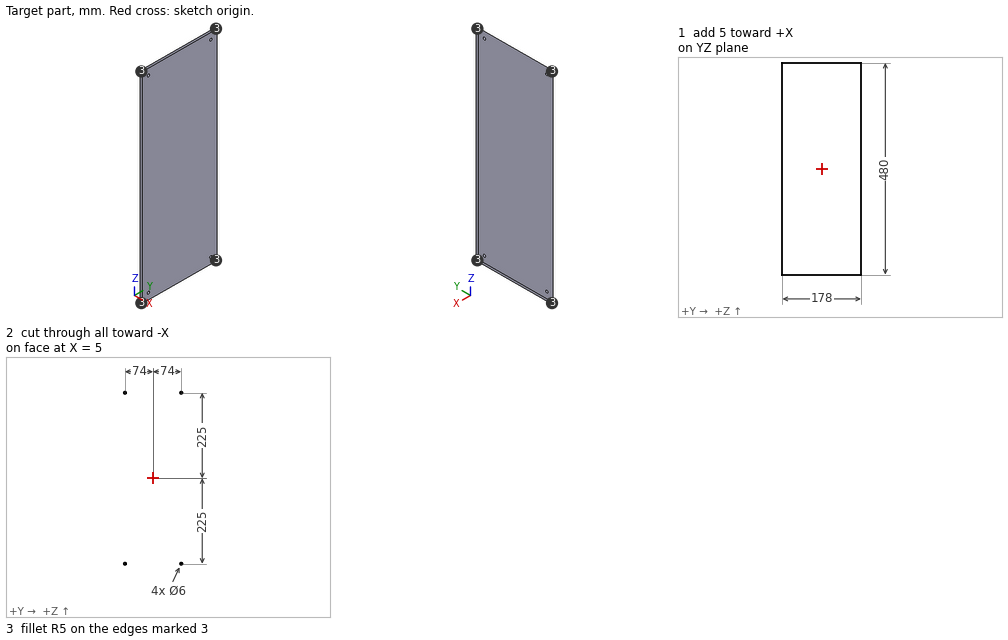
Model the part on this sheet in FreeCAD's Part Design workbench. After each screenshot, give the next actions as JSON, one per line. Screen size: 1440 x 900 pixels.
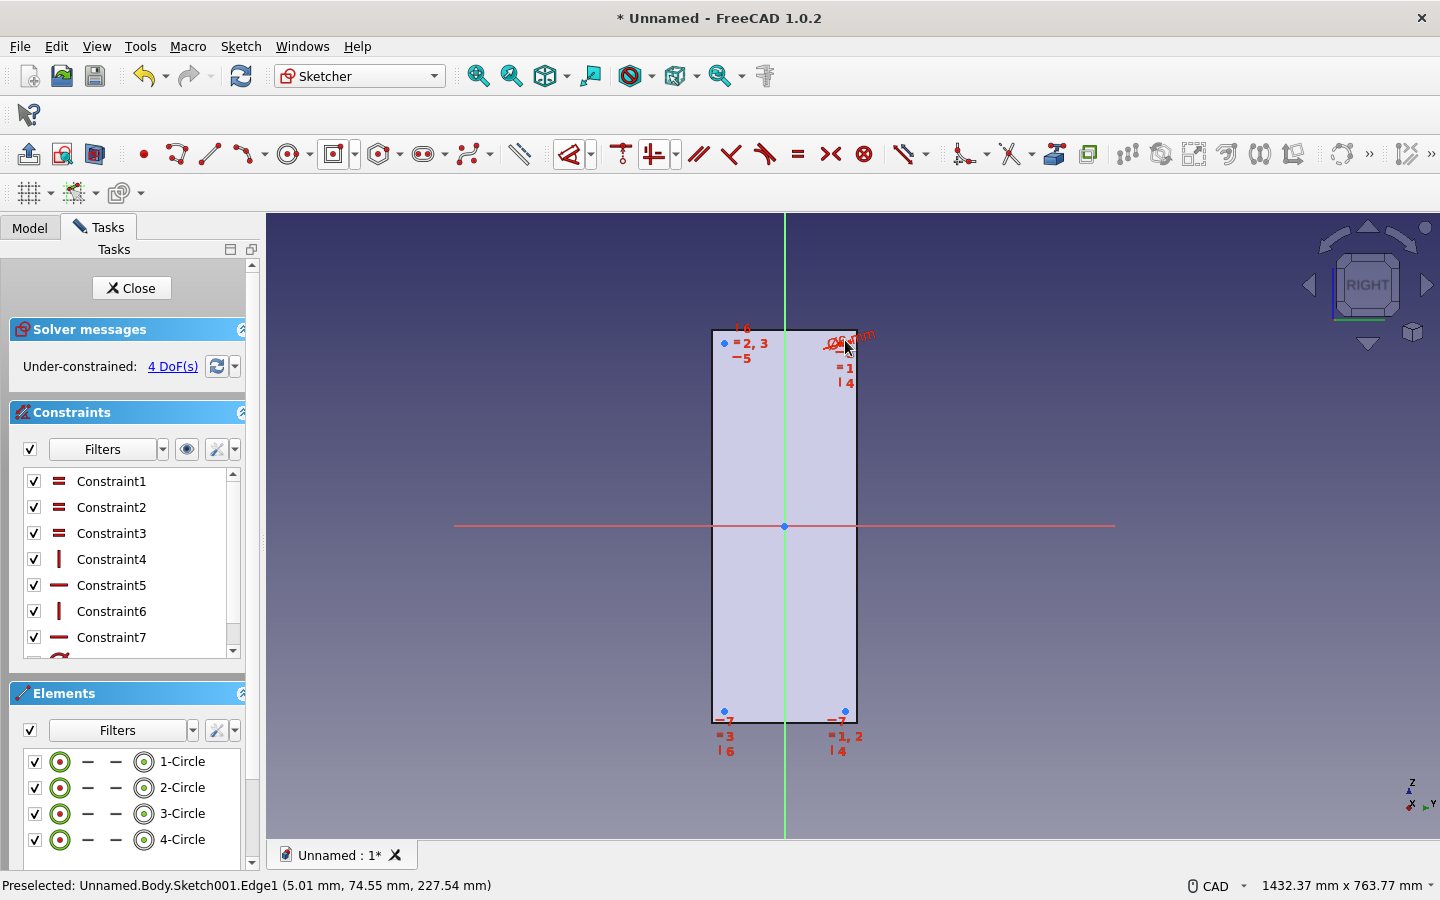
{"action": "left_click", "coordinate": [845, 343]}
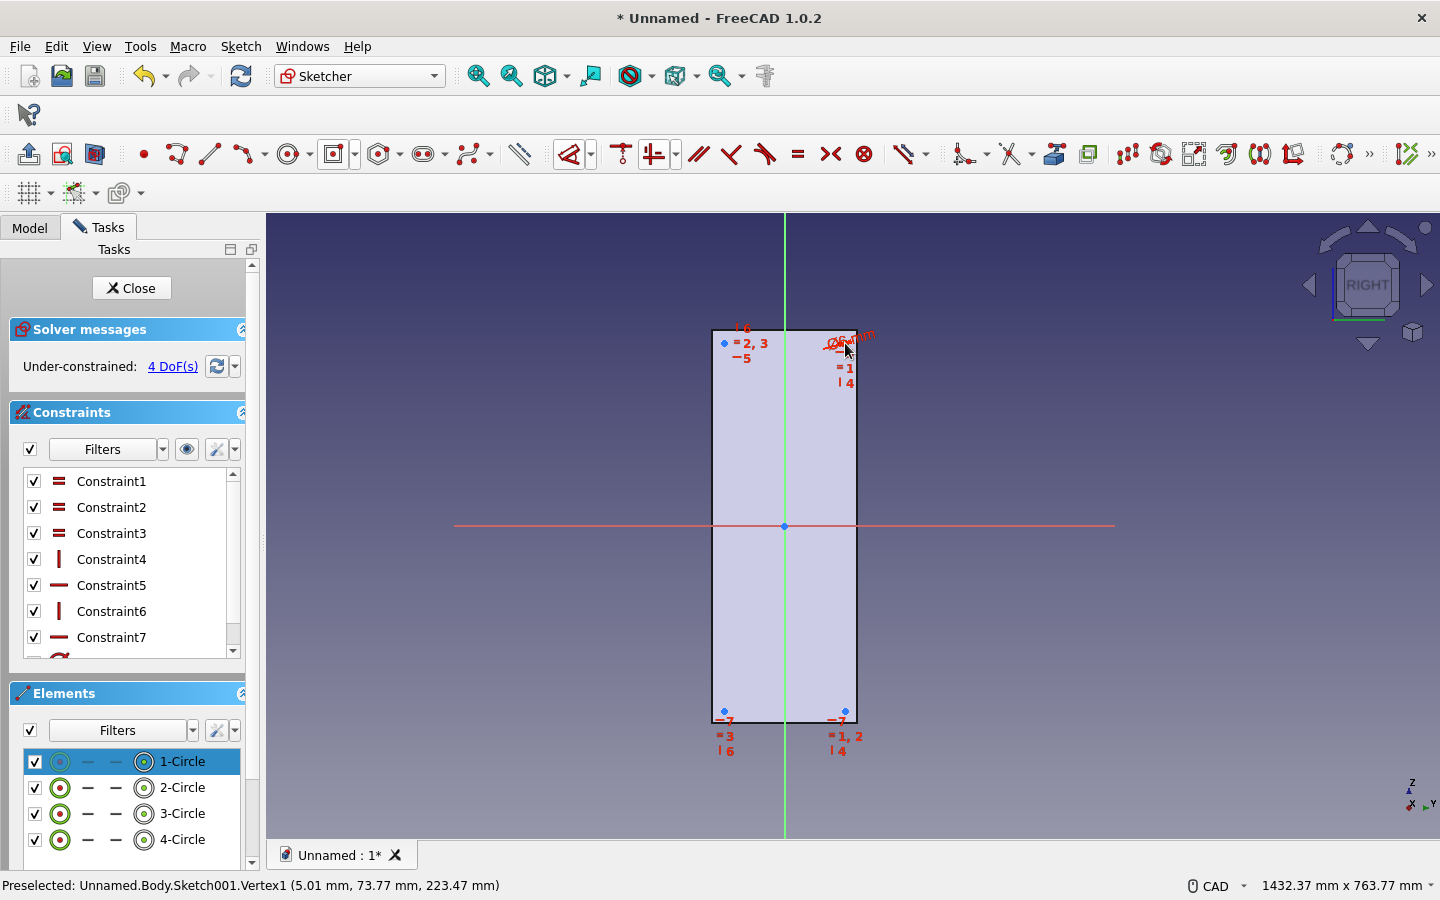
{"action": "left_click", "coordinate": [590, 154]}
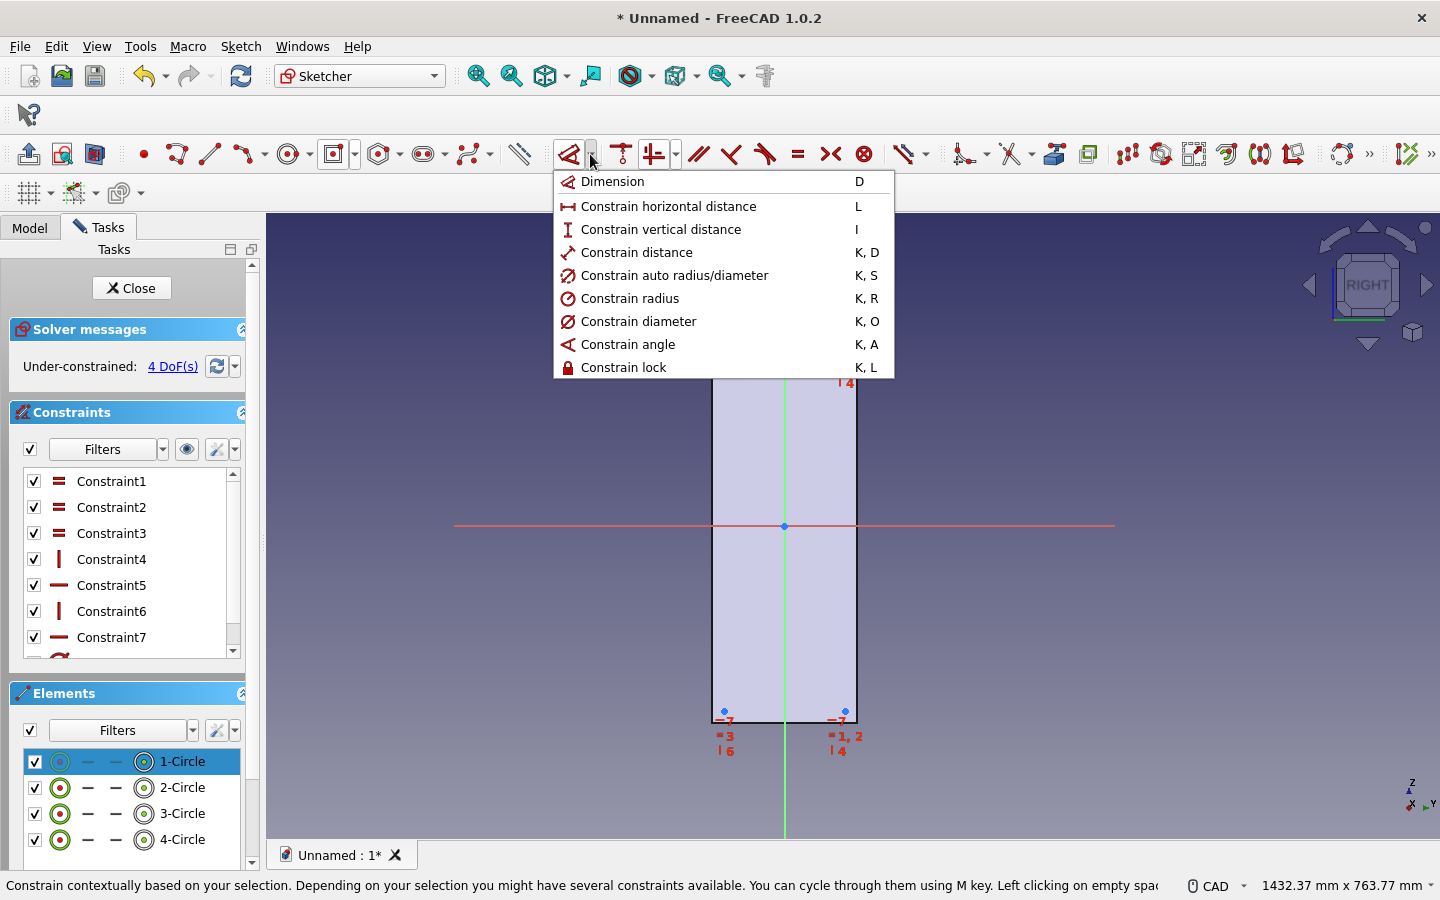
{"action": "left_click", "coordinate": [724, 206]}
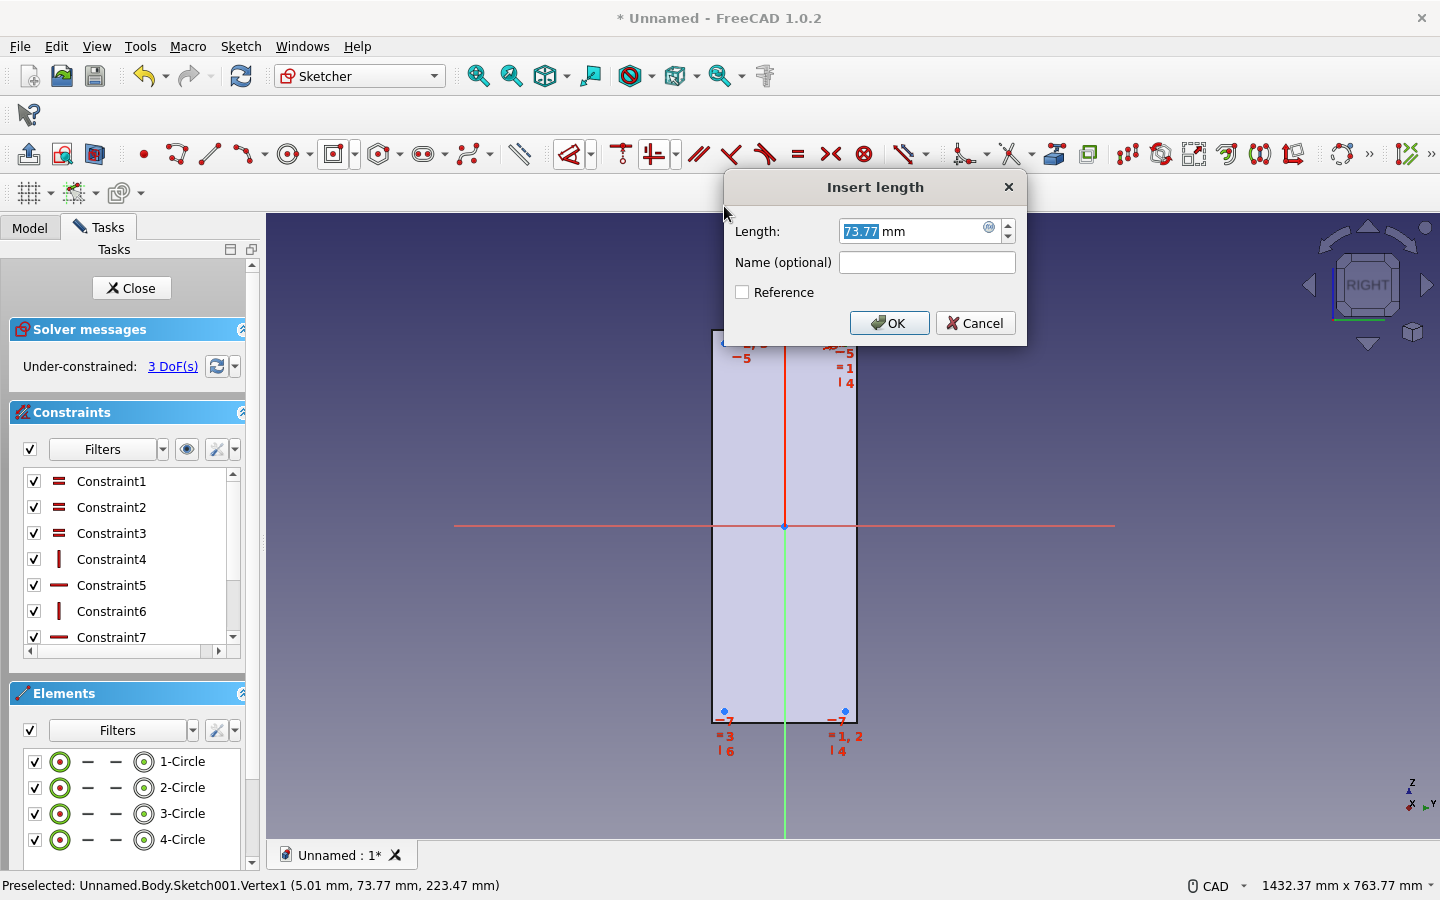
{"action": "type", "text": "74"}
{"action": "key", "text": "Return"}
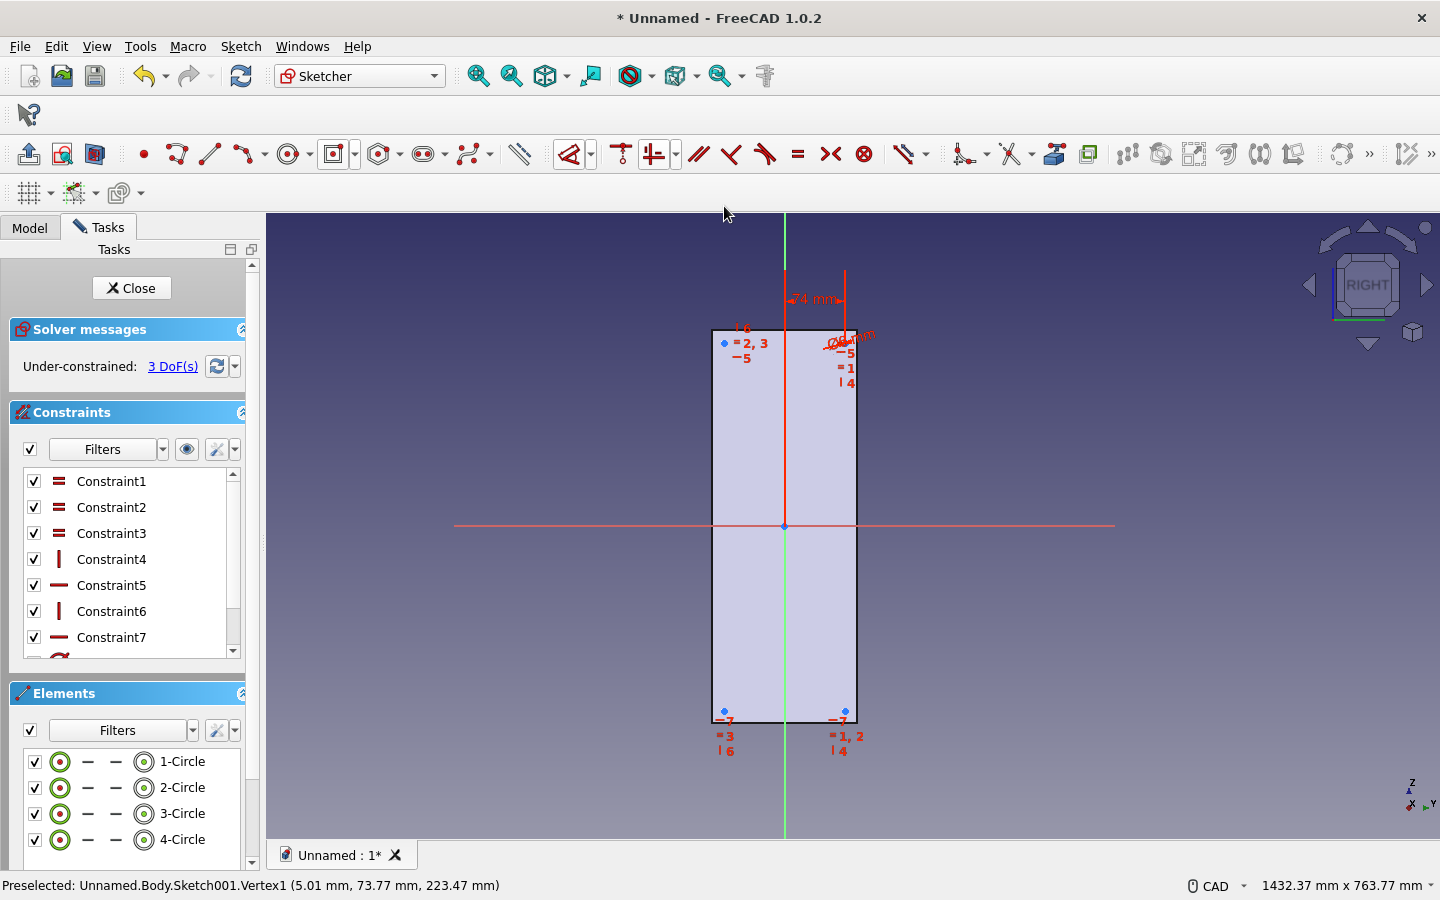
{"action": "left_click", "coordinate": [724, 343]}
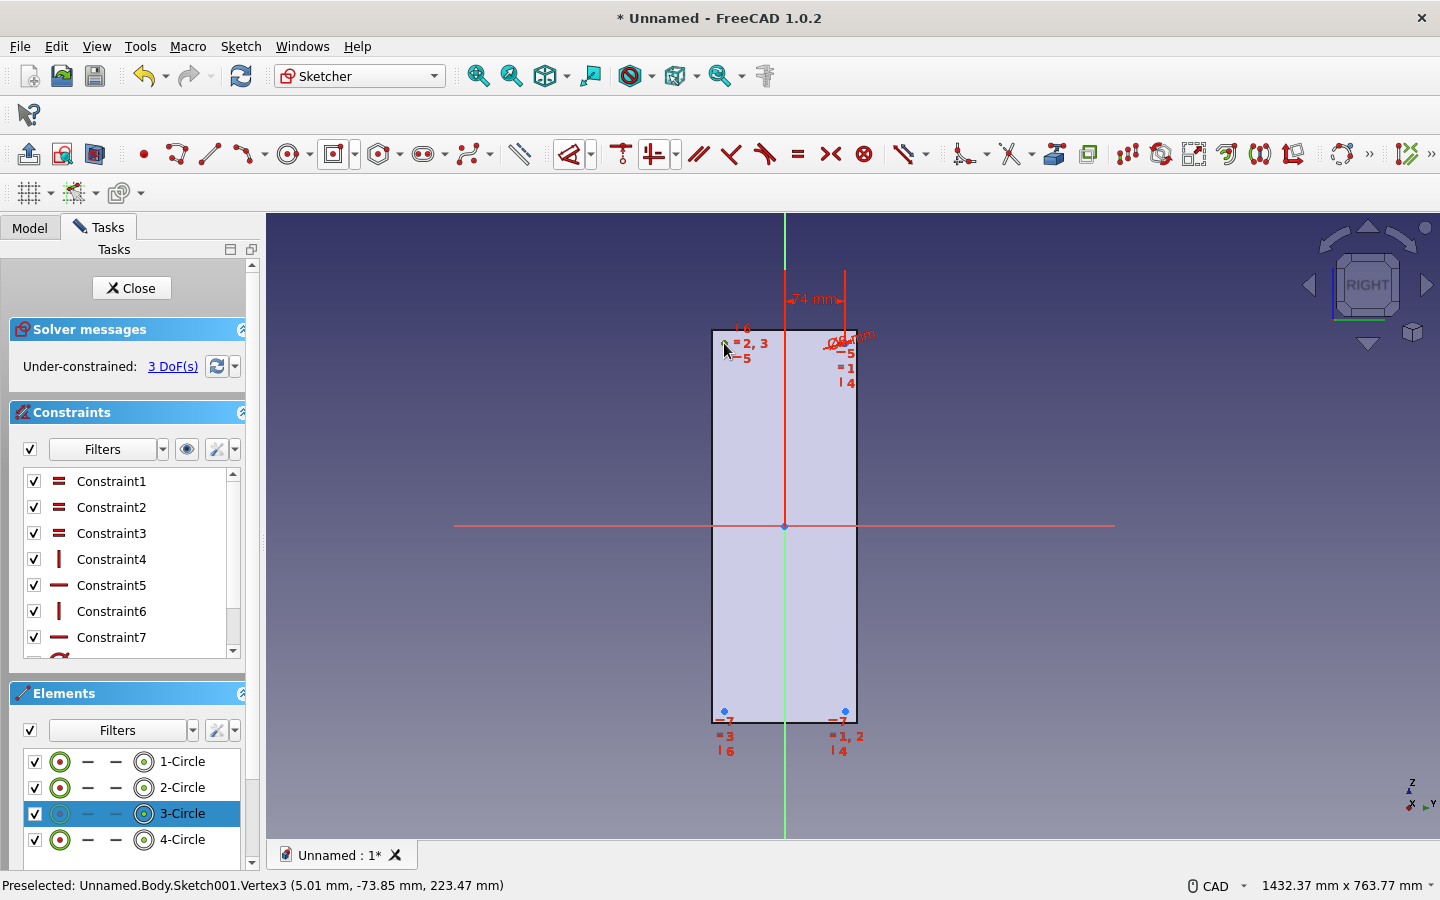
{"action": "key", "text": "l"}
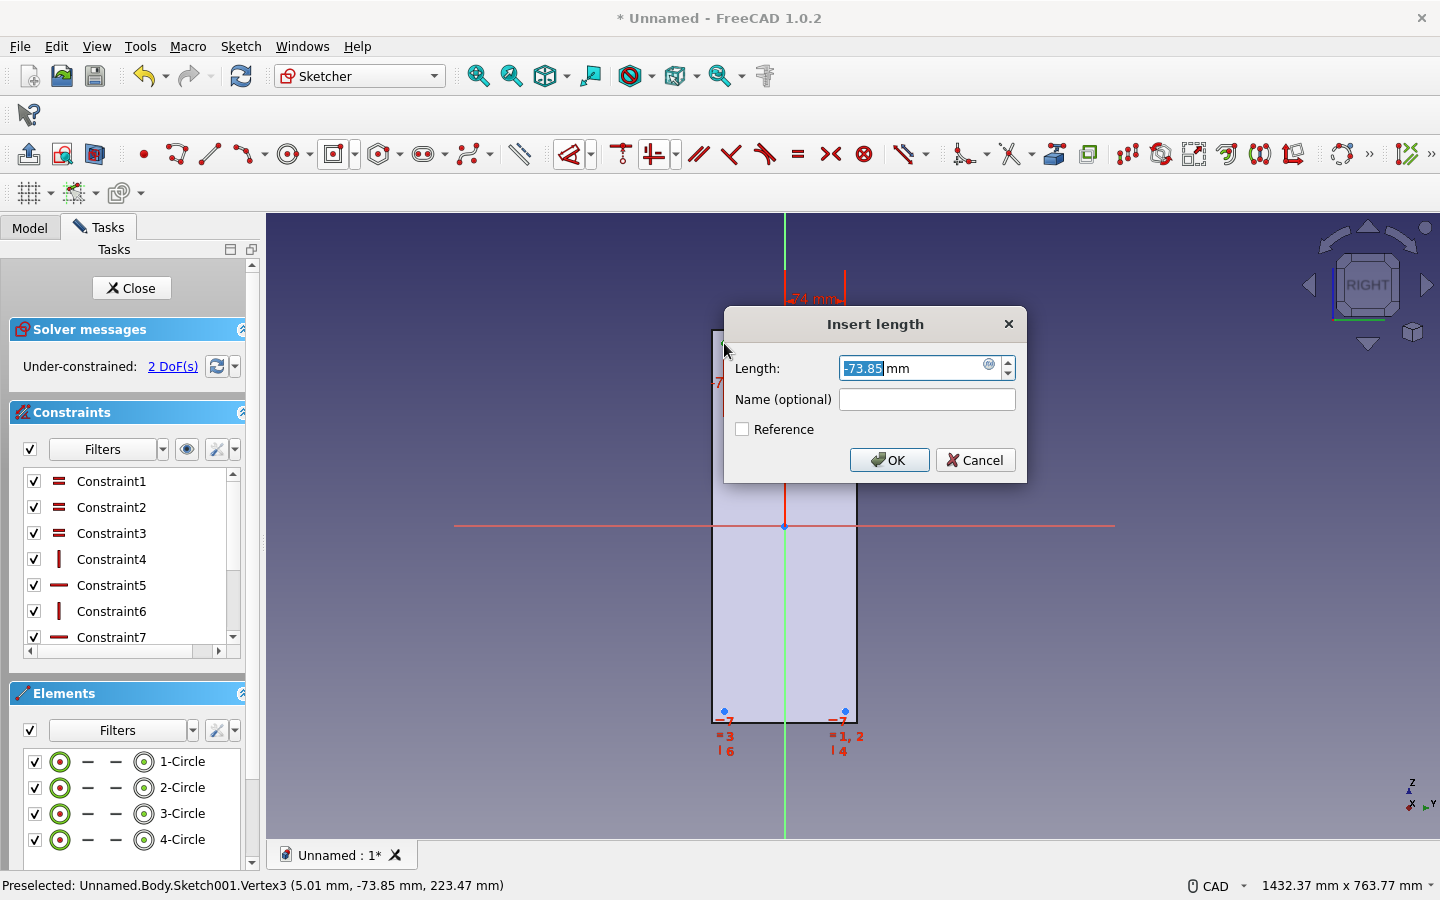
{"action": "type", "text": "-74"}
{"action": "key", "text": "Return"}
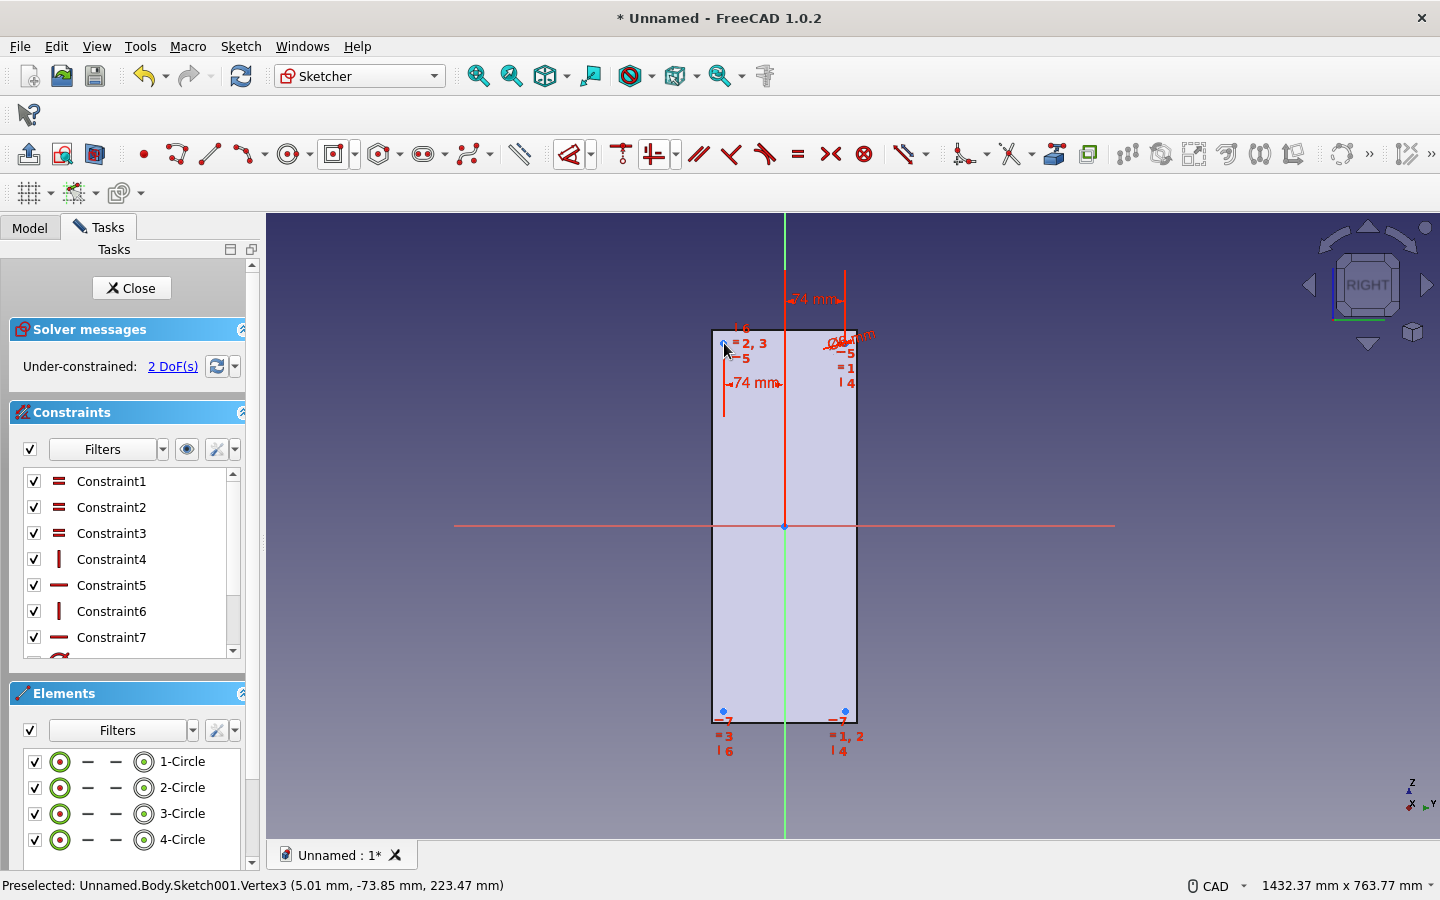
{"action": "left_click", "coordinate": [845, 343]}